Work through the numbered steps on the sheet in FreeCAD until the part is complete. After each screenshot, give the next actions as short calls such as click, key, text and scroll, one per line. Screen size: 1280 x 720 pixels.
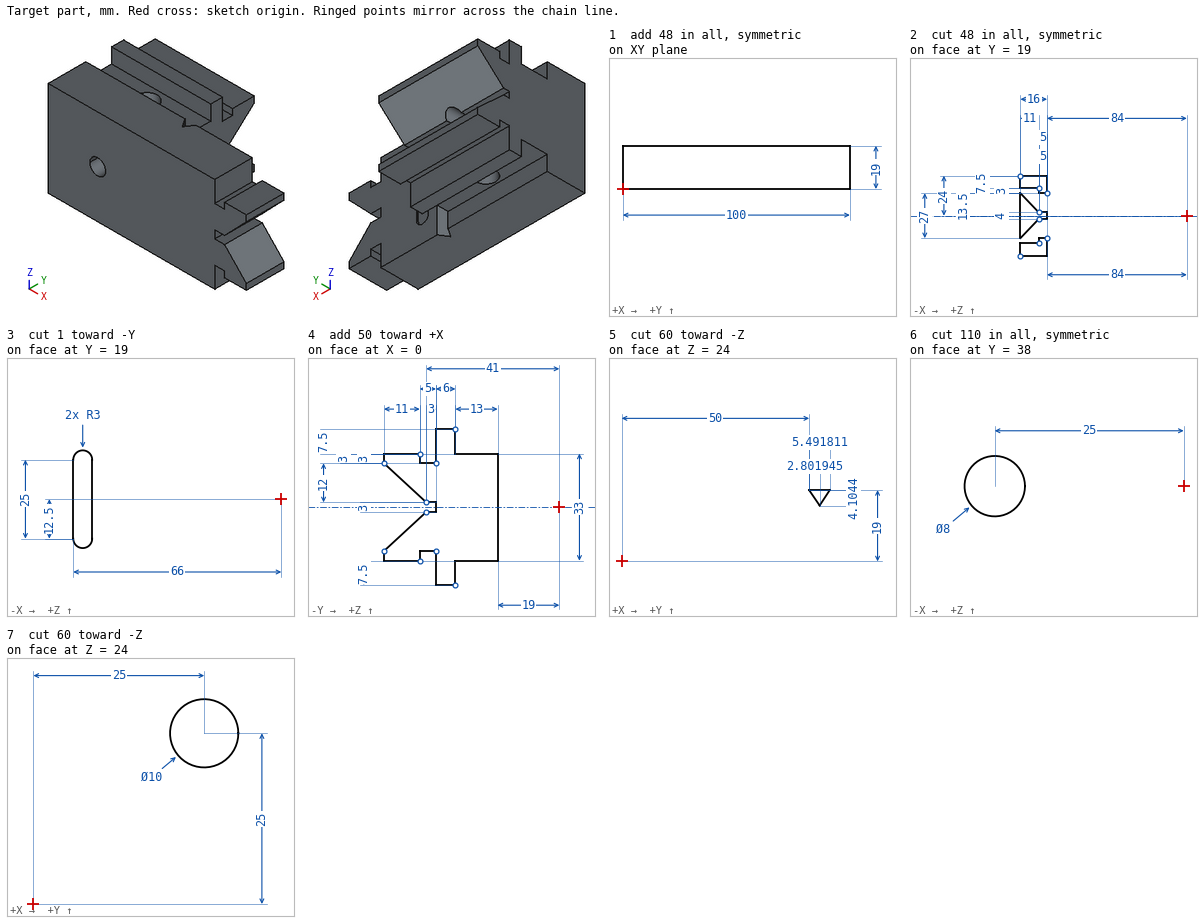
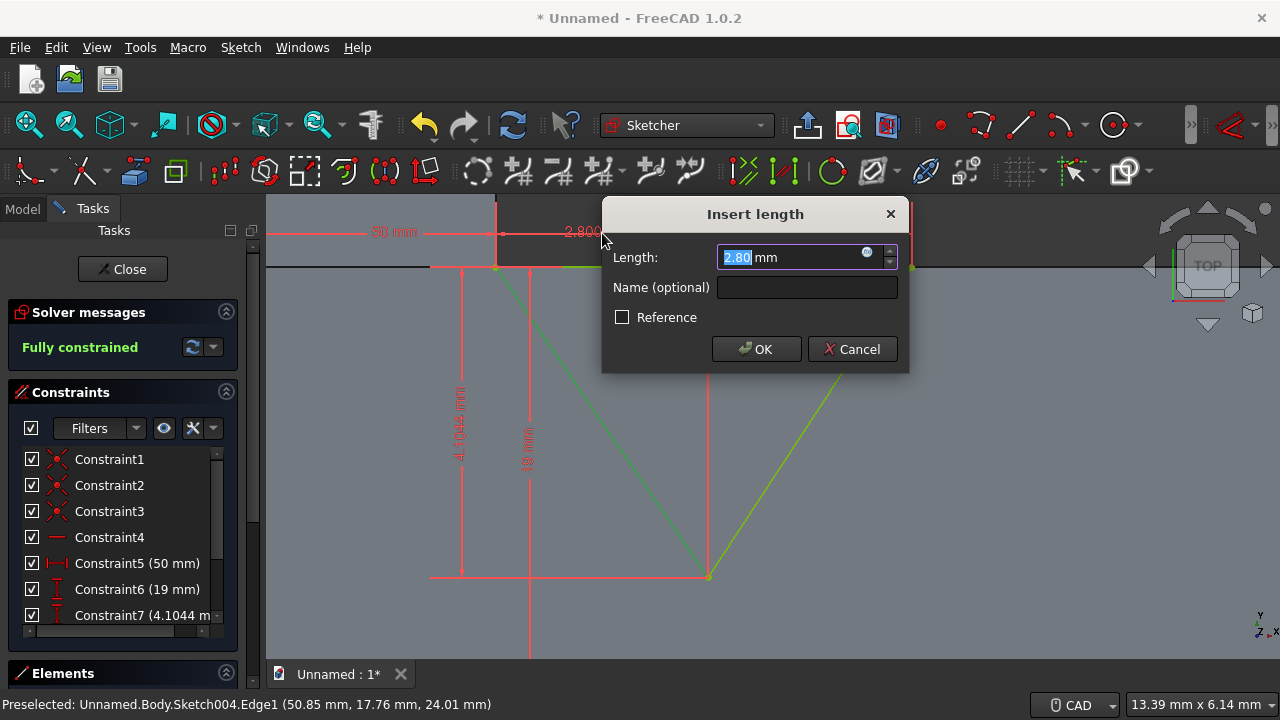
text(2.801945)
key(Return)
key(Escape)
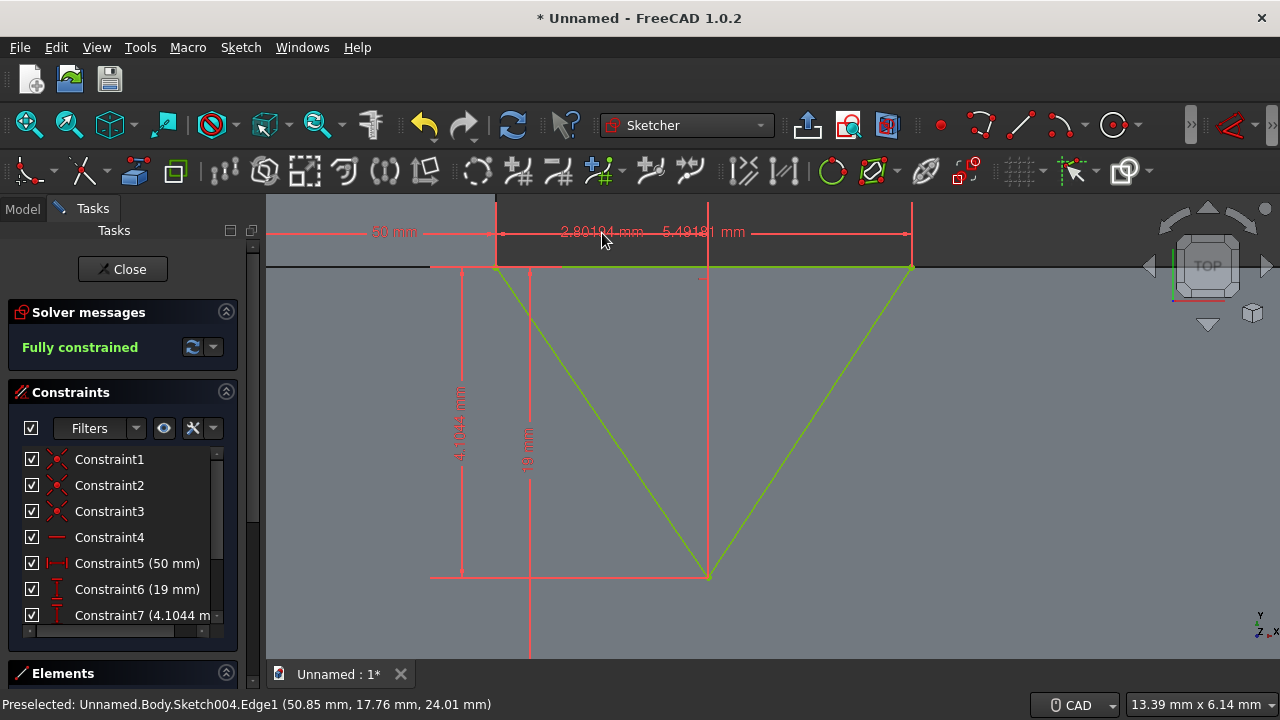
click(123, 269)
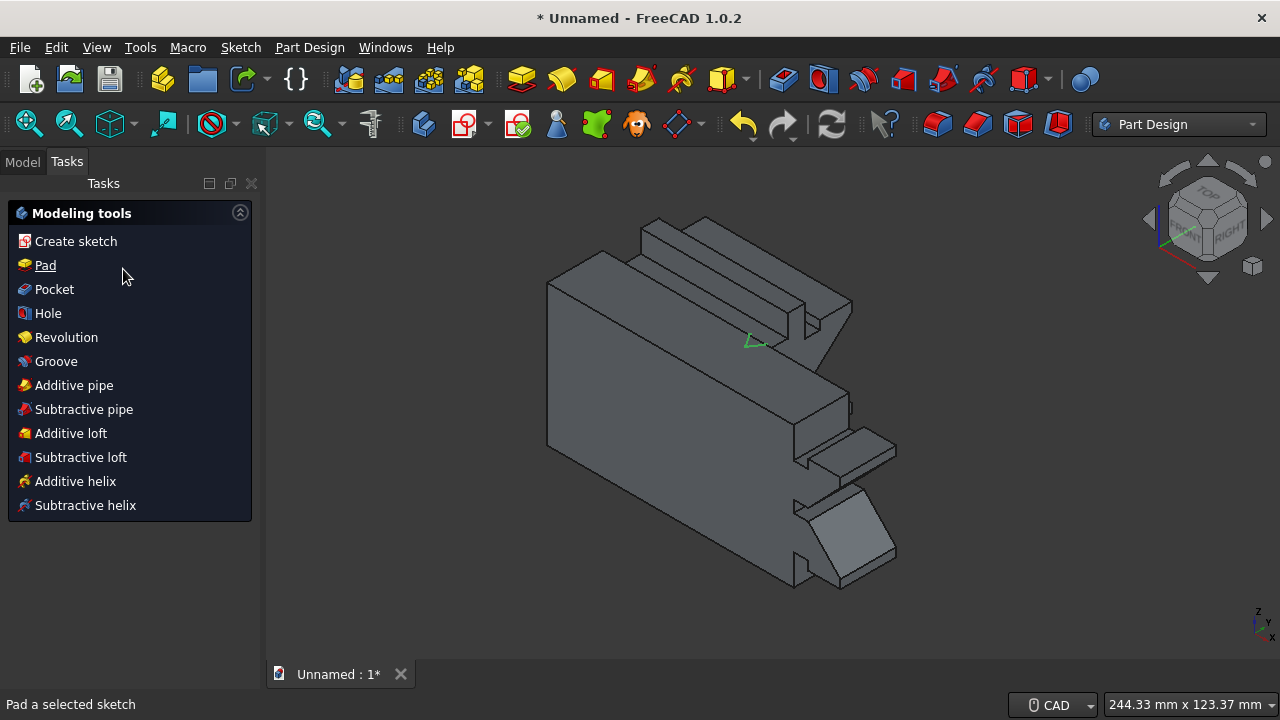
click(784, 80)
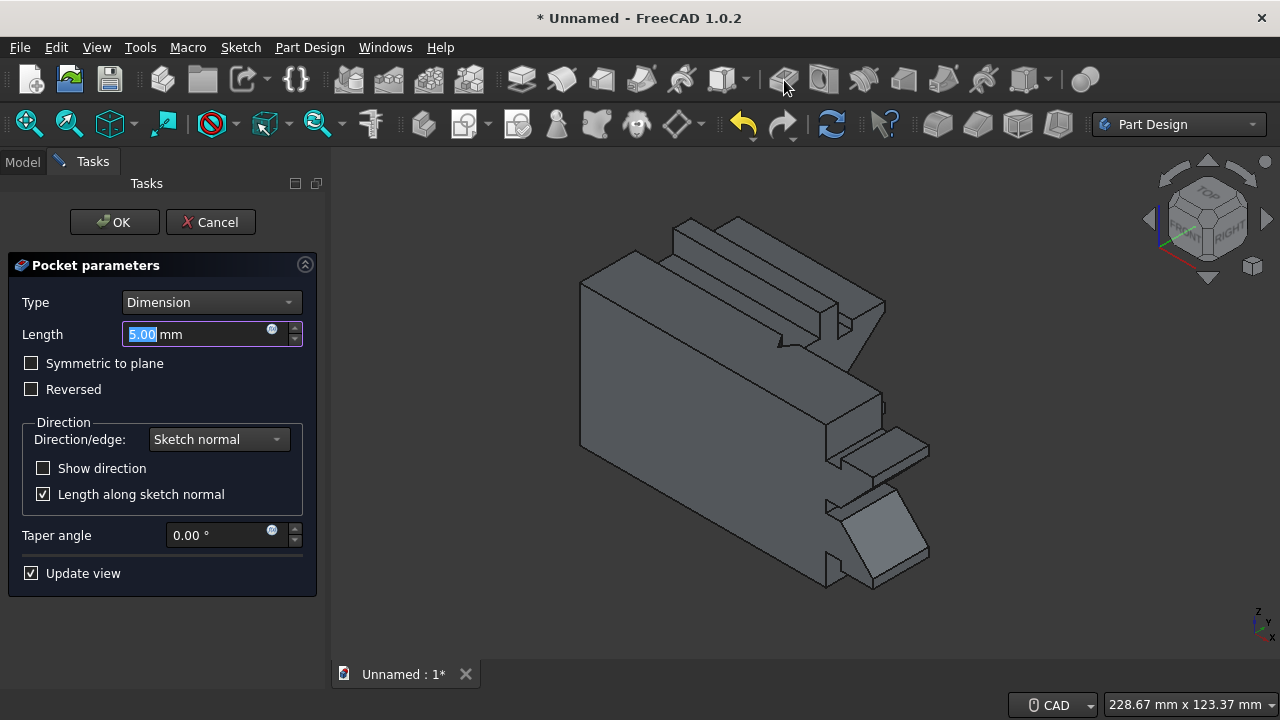
text(60)
key(Tab)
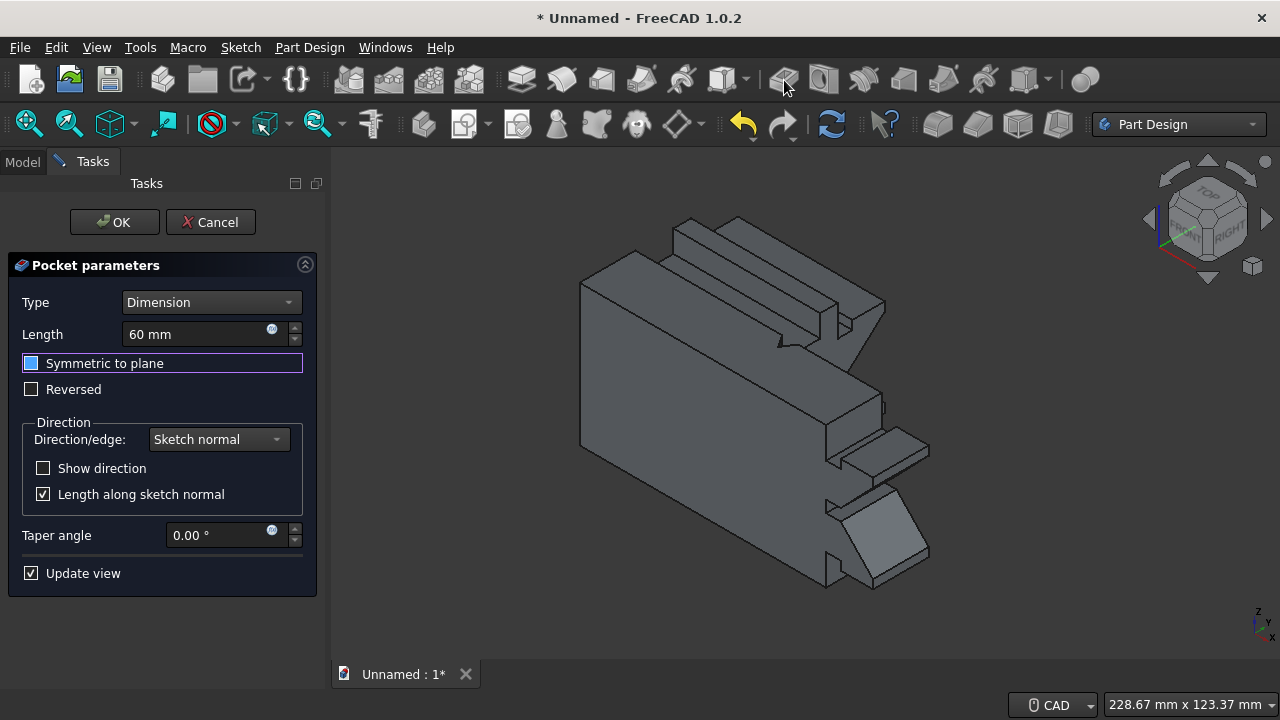
click(115, 222)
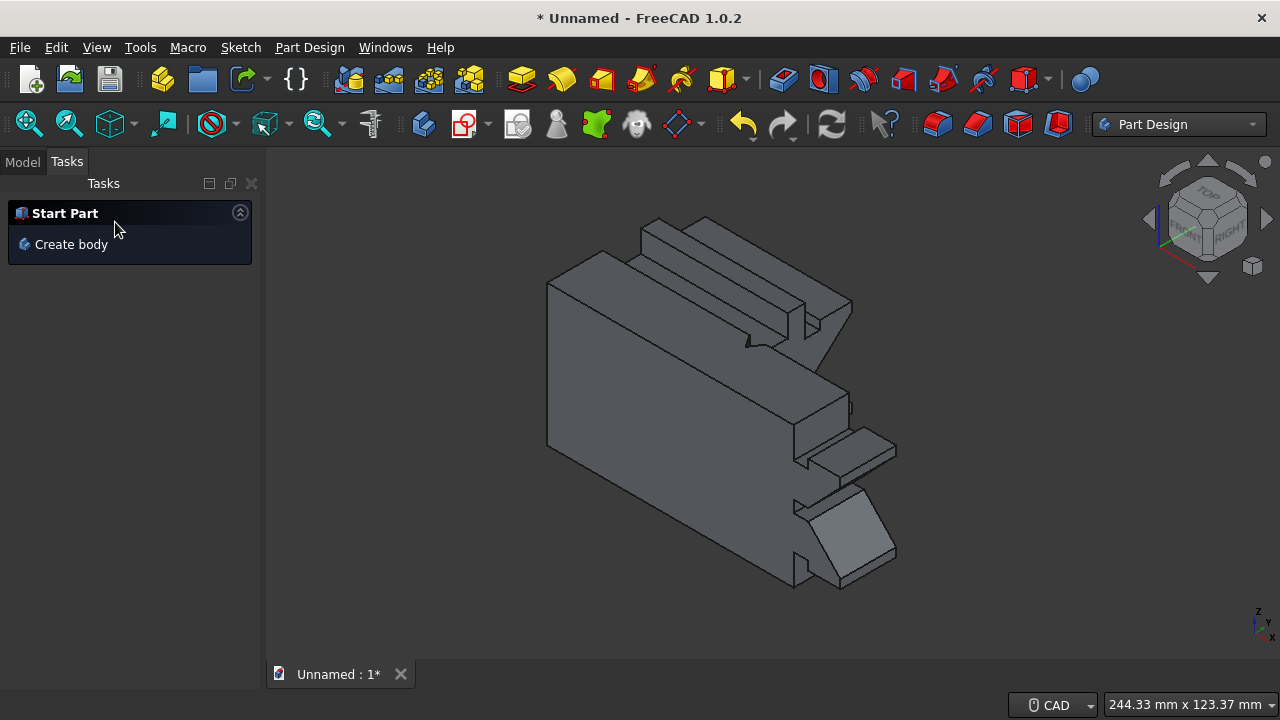
key(4)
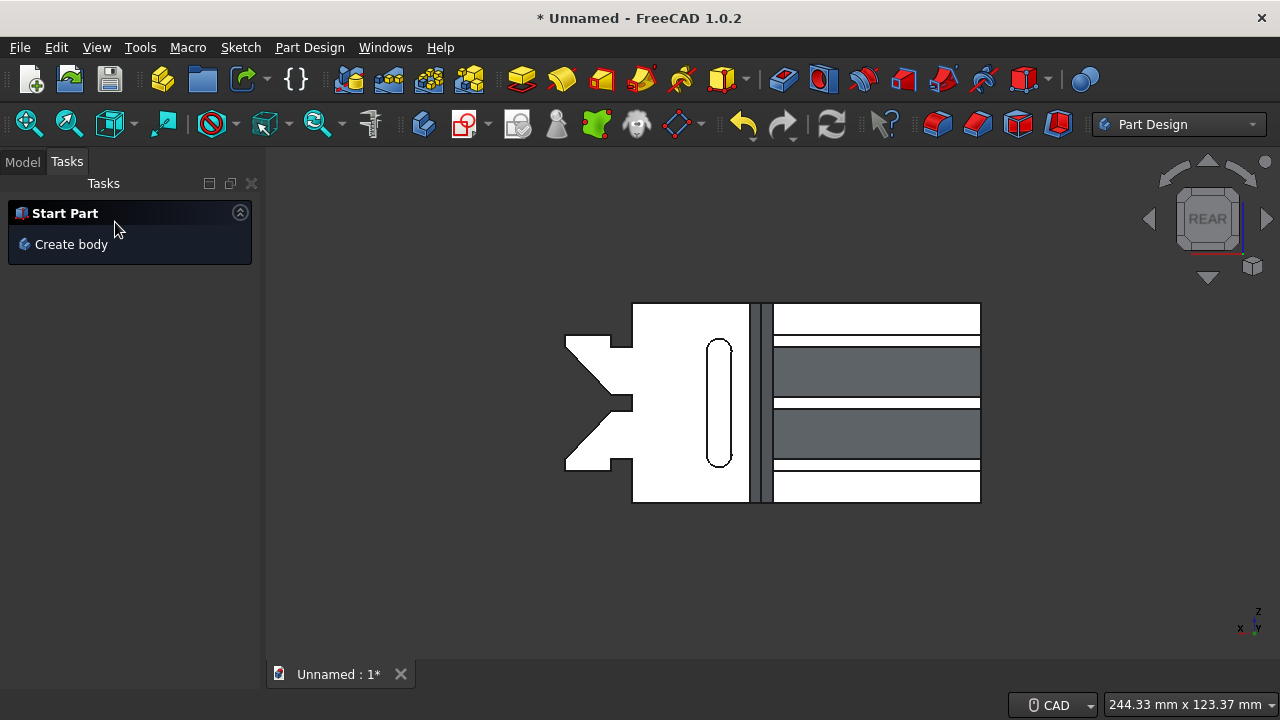
click(30, 124)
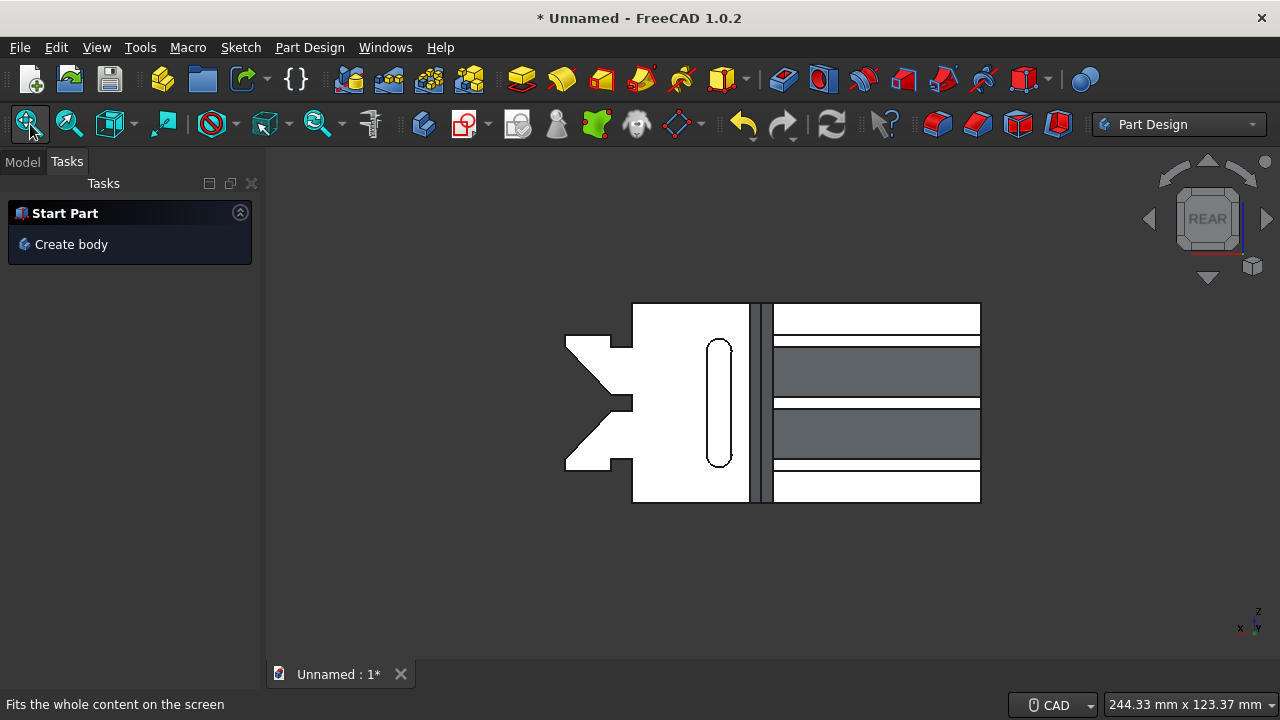
click(817, 480)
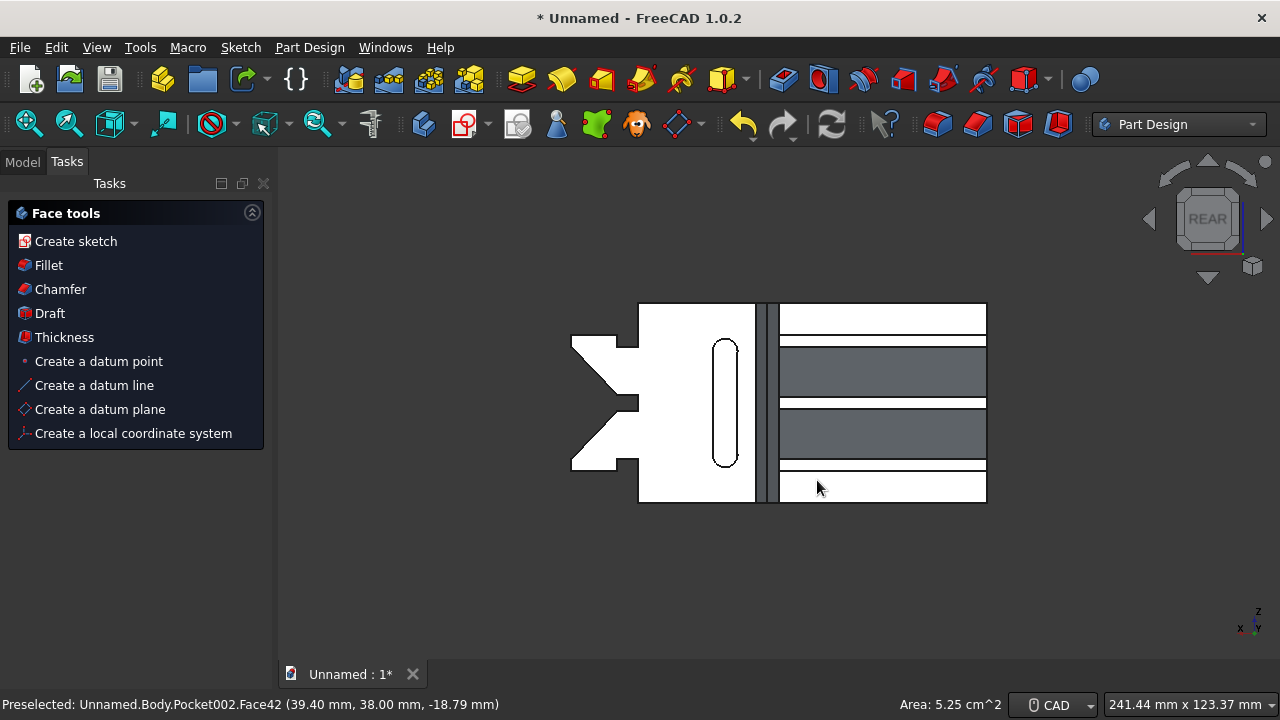
click(464, 124)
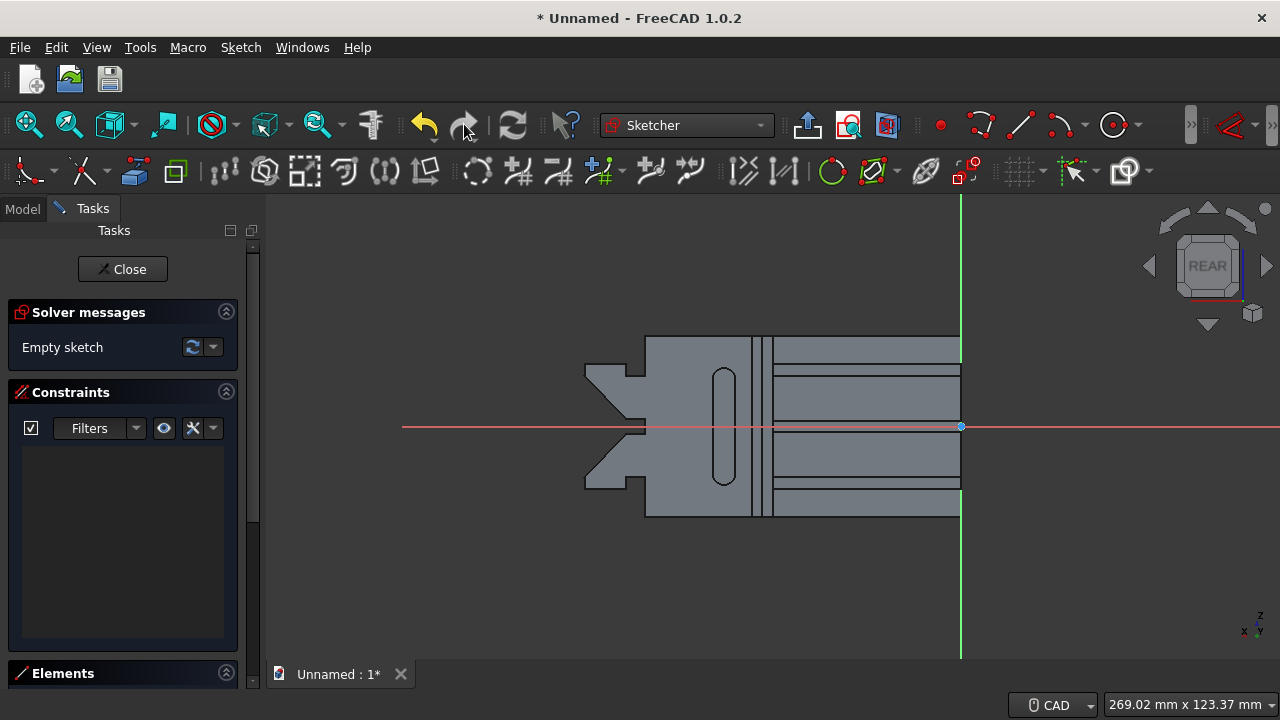
scroll(888, 426, up, 11)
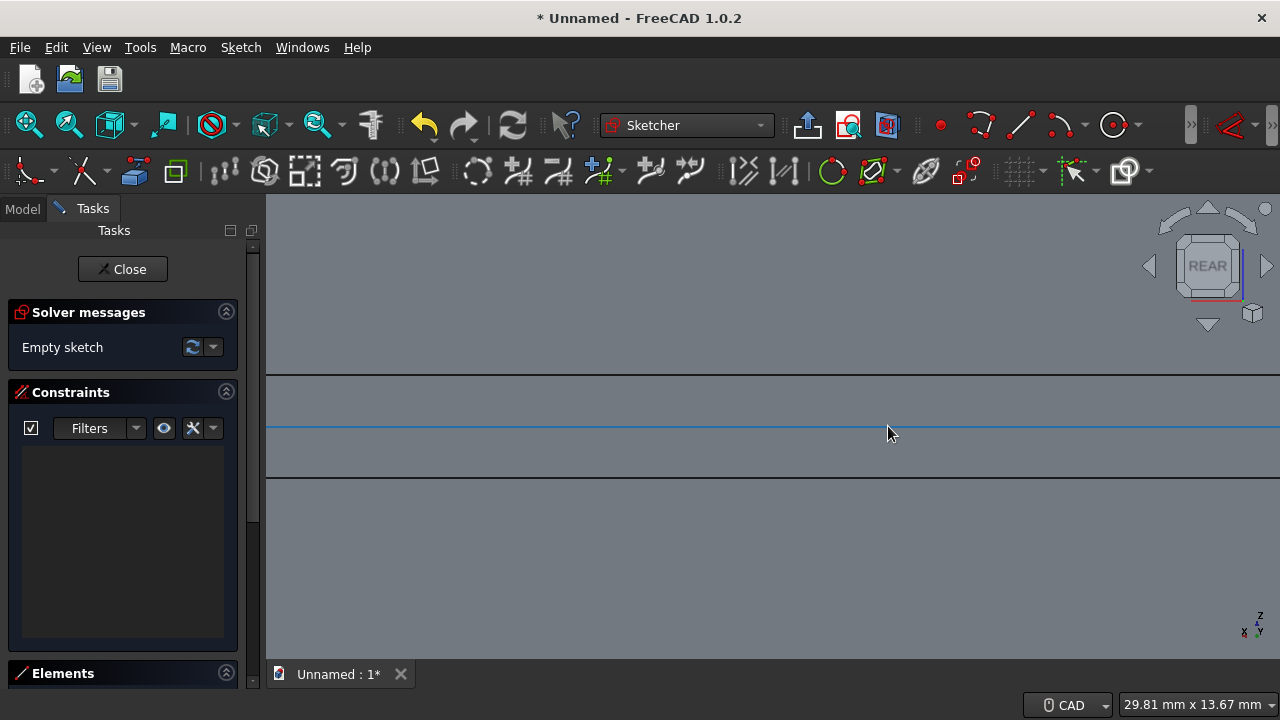
click(1114, 126)